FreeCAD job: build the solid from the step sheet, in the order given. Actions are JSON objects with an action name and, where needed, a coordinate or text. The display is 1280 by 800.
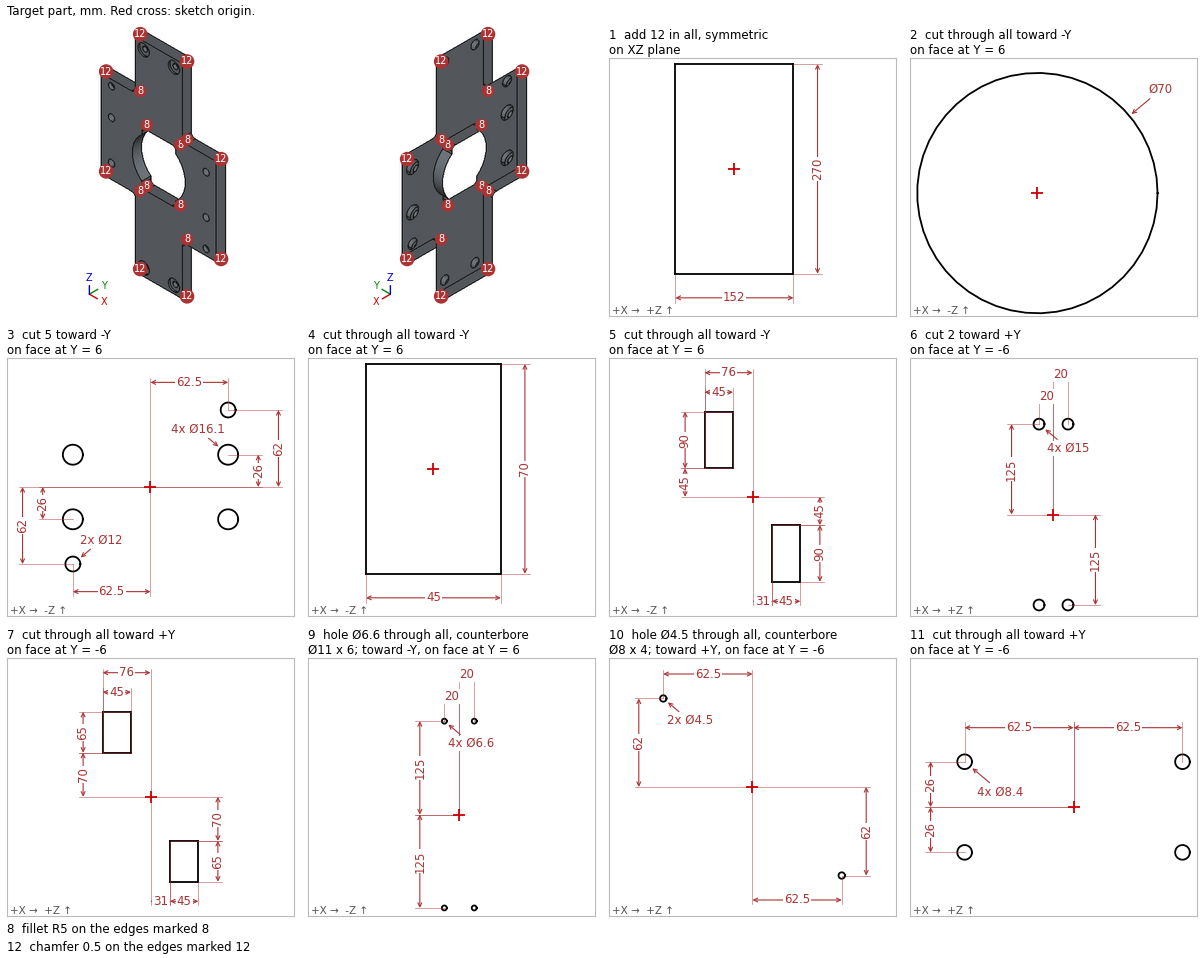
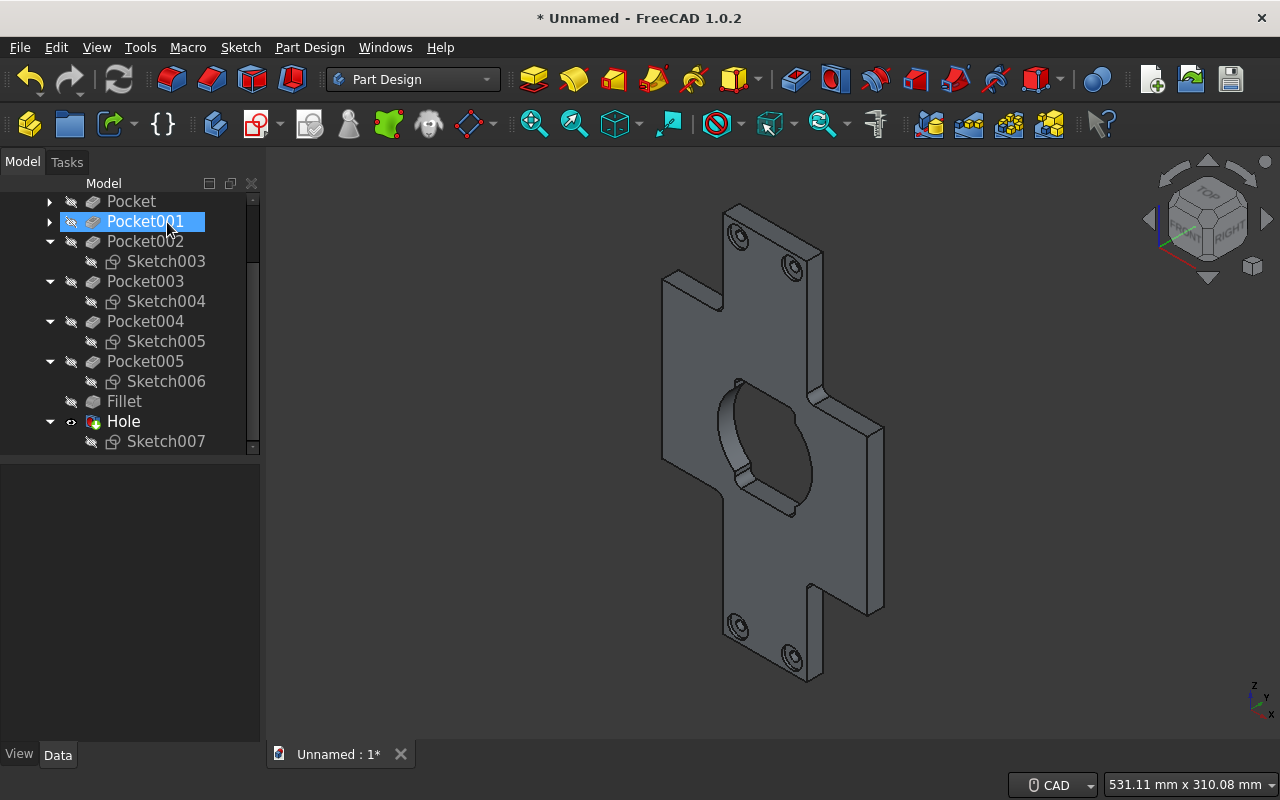
{"action": "left_click", "coordinate": [765, 326]}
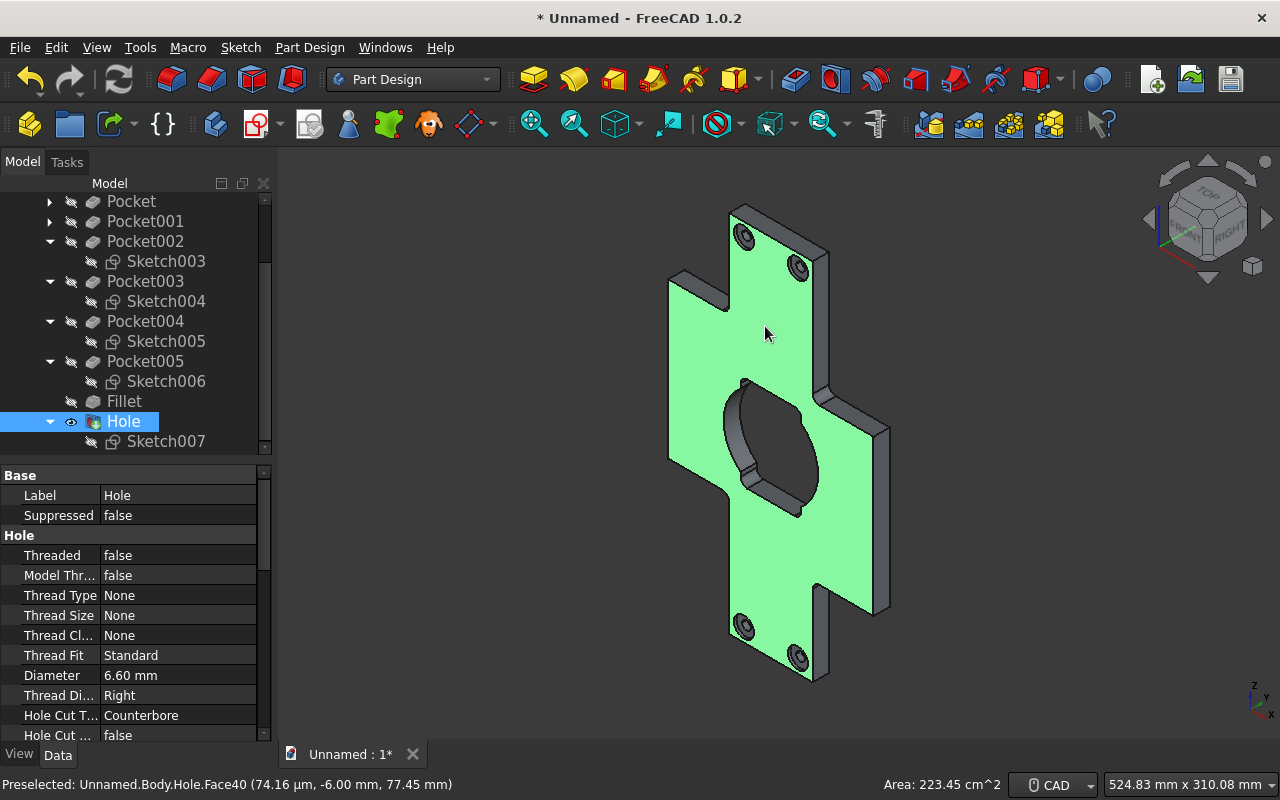
{"action": "left_click", "coordinate": [256, 124]}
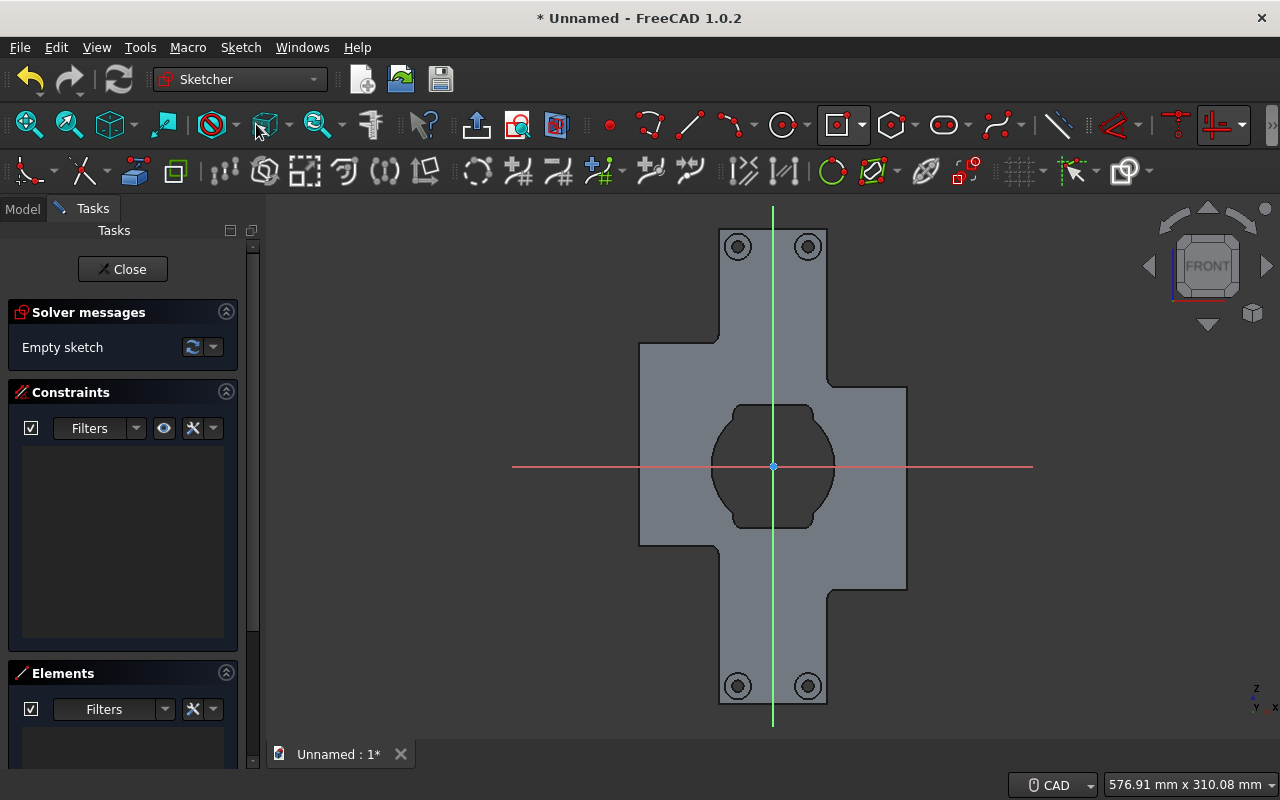
{"action": "scroll", "coordinate": [912, 466], "scroll_direction": "up", "scroll_amount": 2}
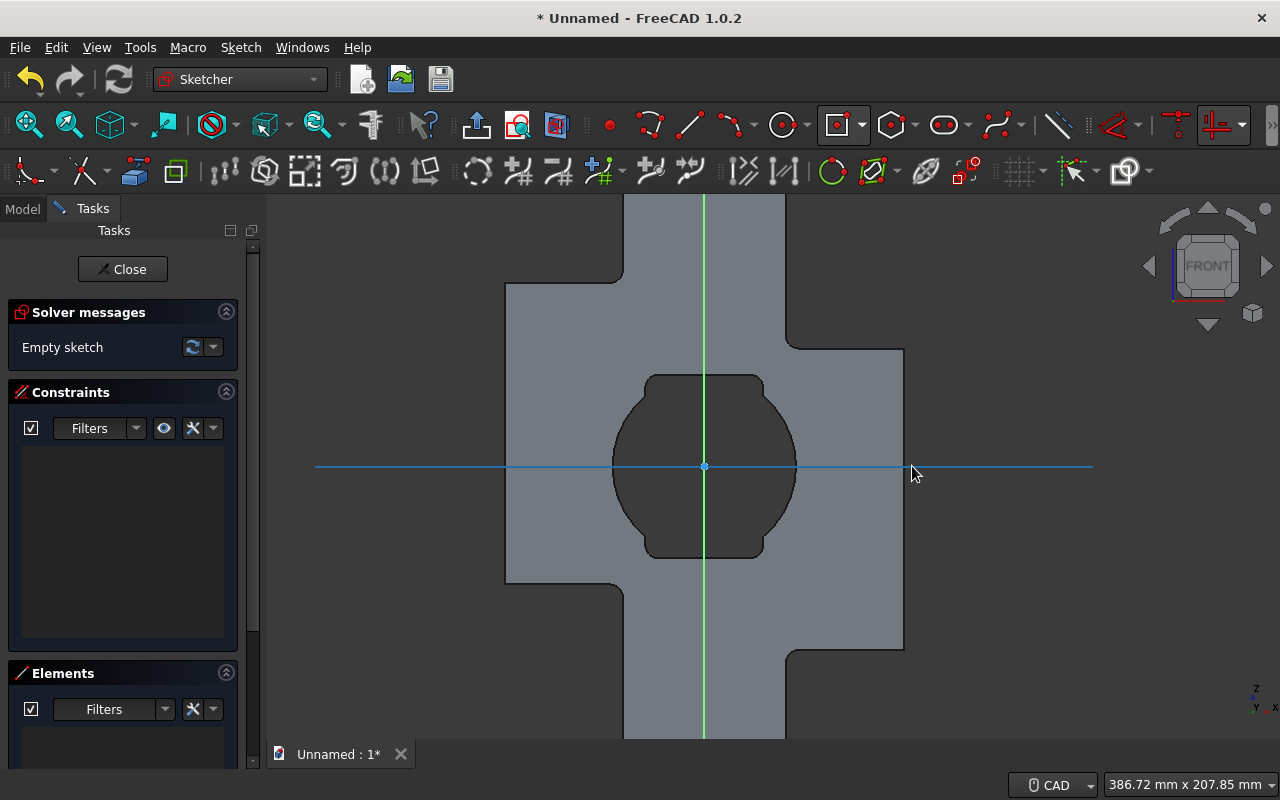
{"action": "key", "text": "g c"}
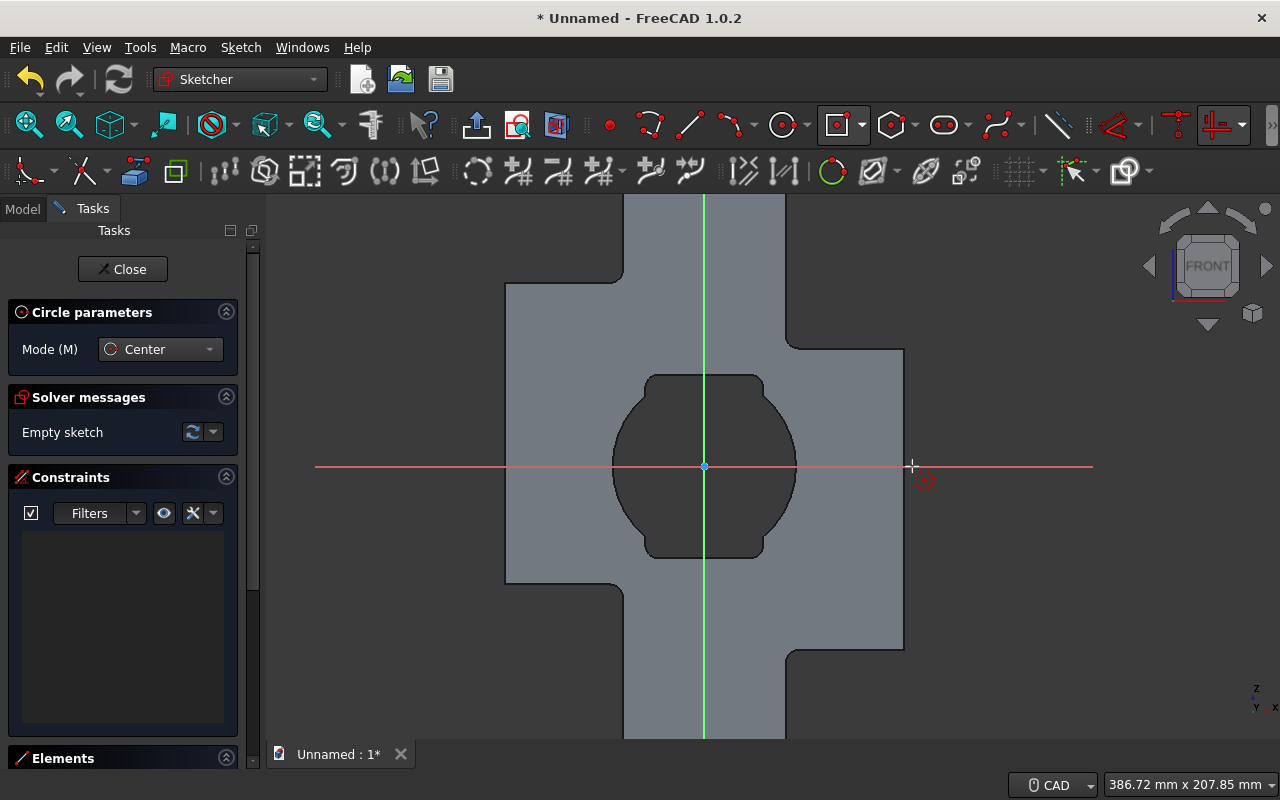
{"action": "scroll", "coordinate": [540, 304], "scroll_direction": "up", "scroll_amount": 7}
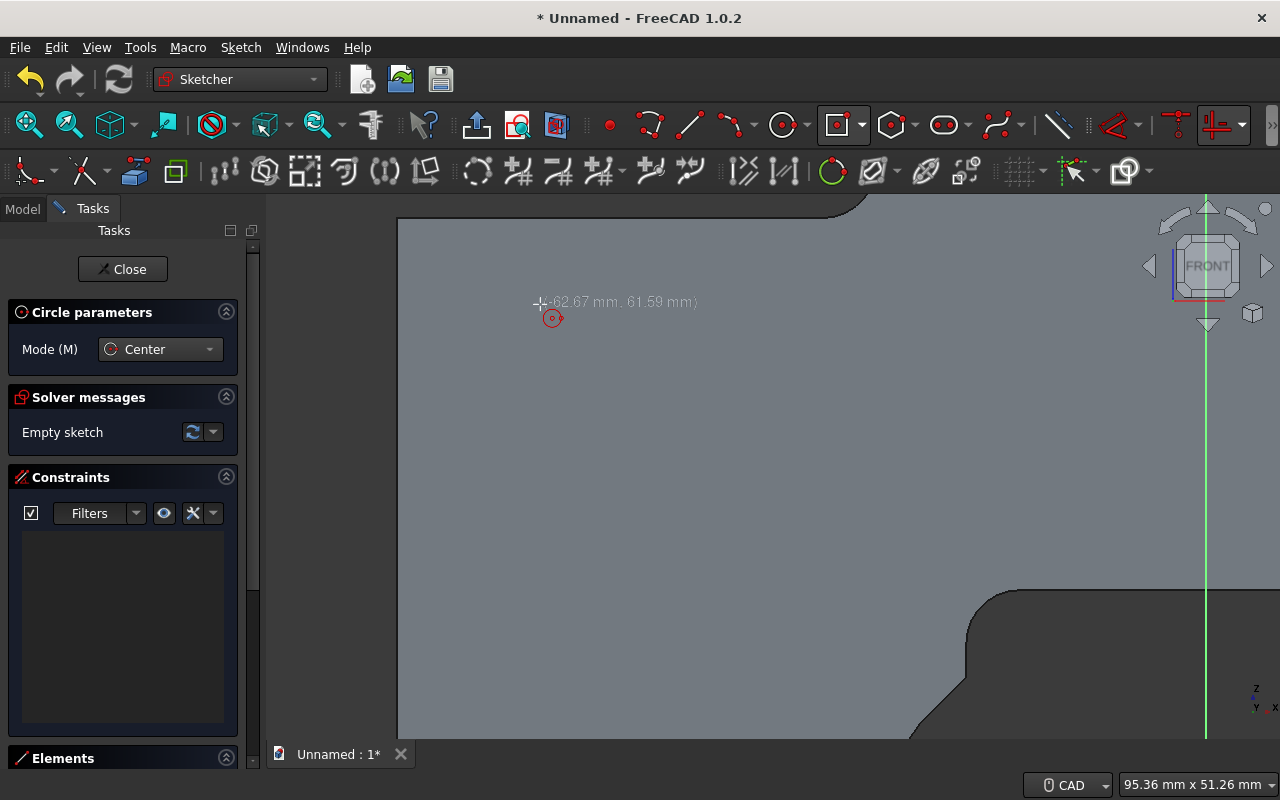
{"action": "scroll", "coordinate": [541, 304], "scroll_direction": "down", "scroll_amount": 7}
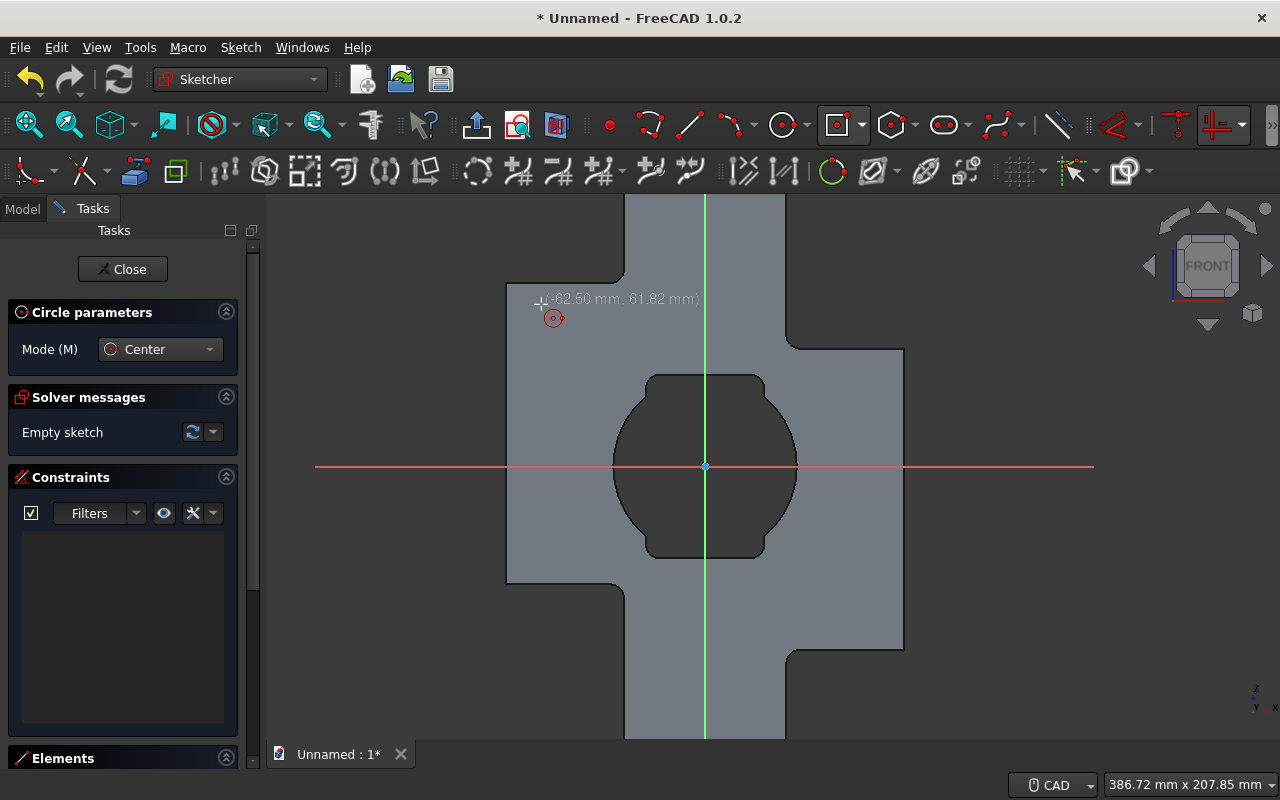
{"action": "left_click", "coordinate": [541, 304]}
{"action": "mouse_move", "coordinate": [545, 300]}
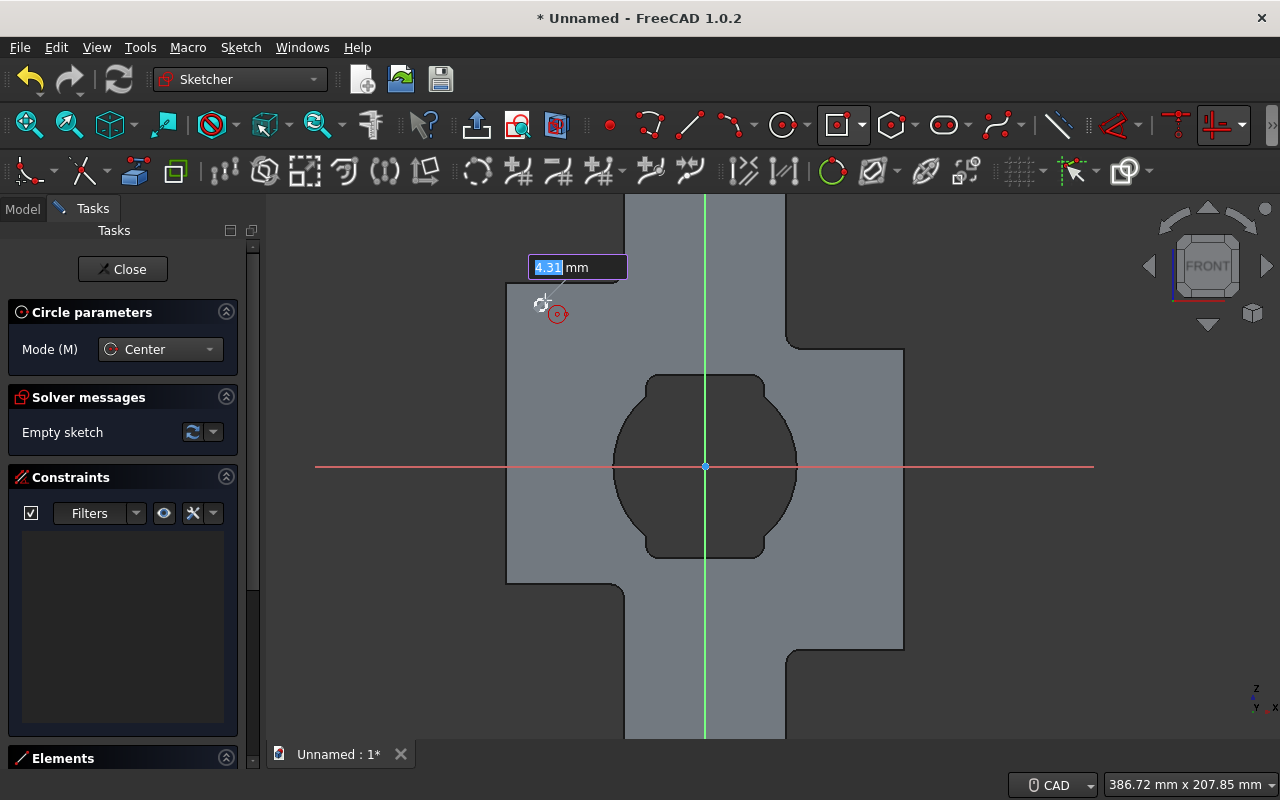
{"action": "type", "text": "4.5"}
{"action": "key", "text": "Return"}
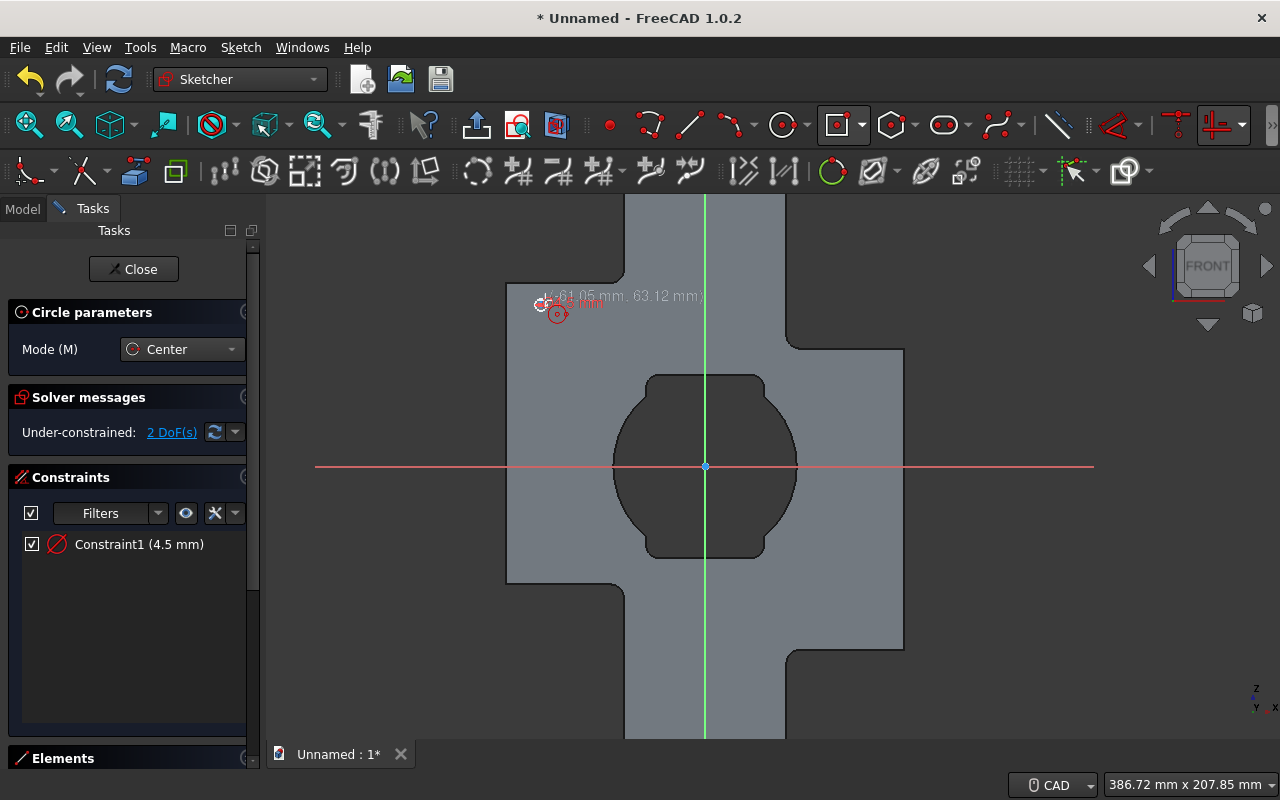
{"action": "scroll", "coordinate": [869, 629], "scroll_direction": "up", "scroll_amount": 7}